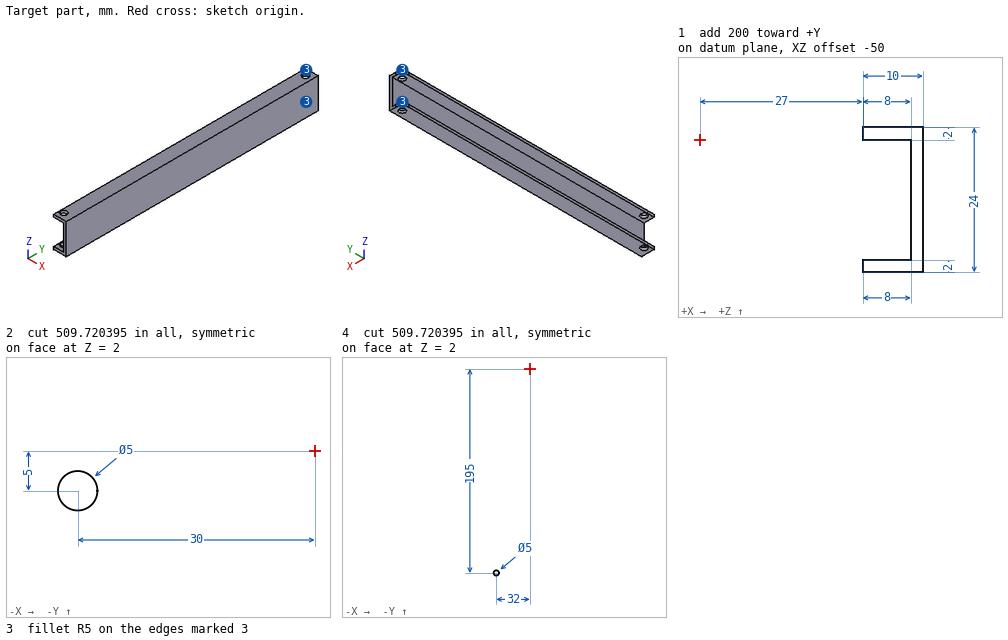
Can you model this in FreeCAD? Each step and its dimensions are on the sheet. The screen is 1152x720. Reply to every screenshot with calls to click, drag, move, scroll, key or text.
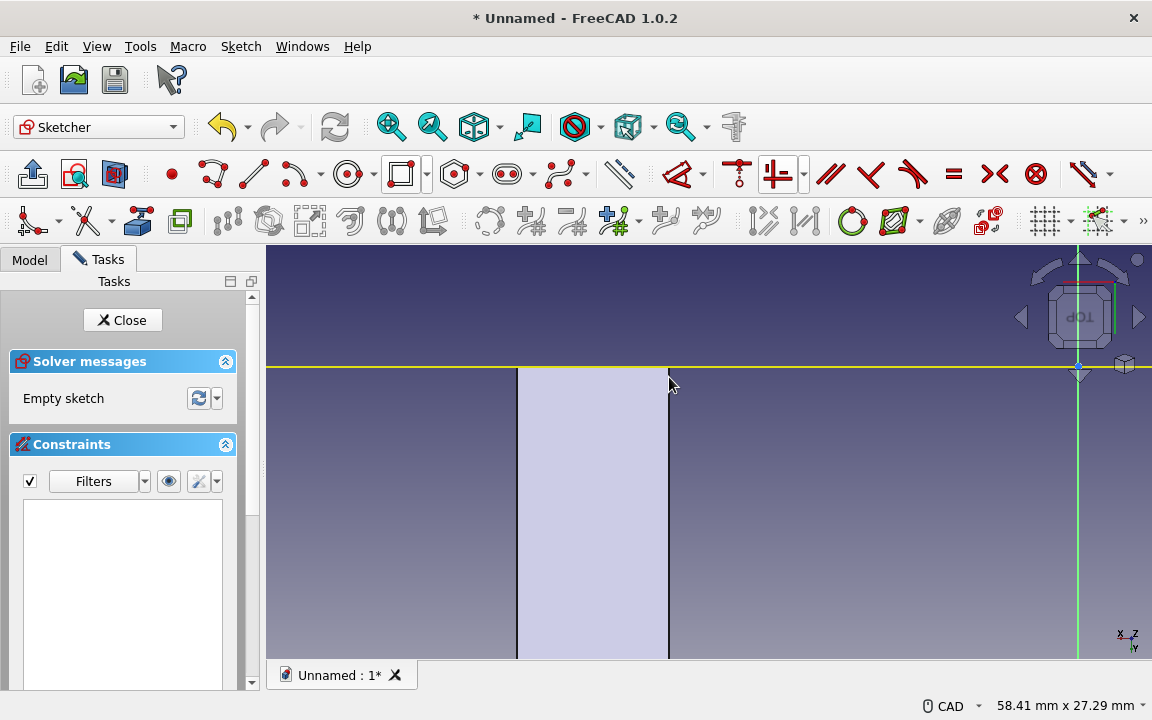
scroll(616, 439, up, 6)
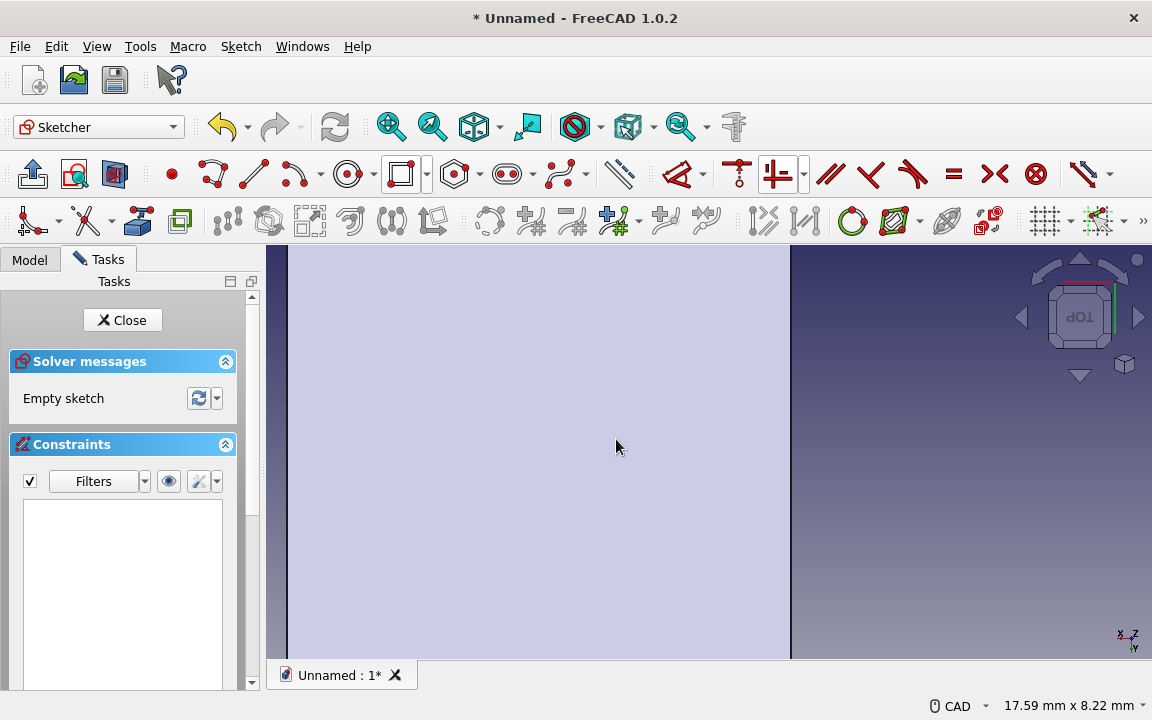
click(348, 174)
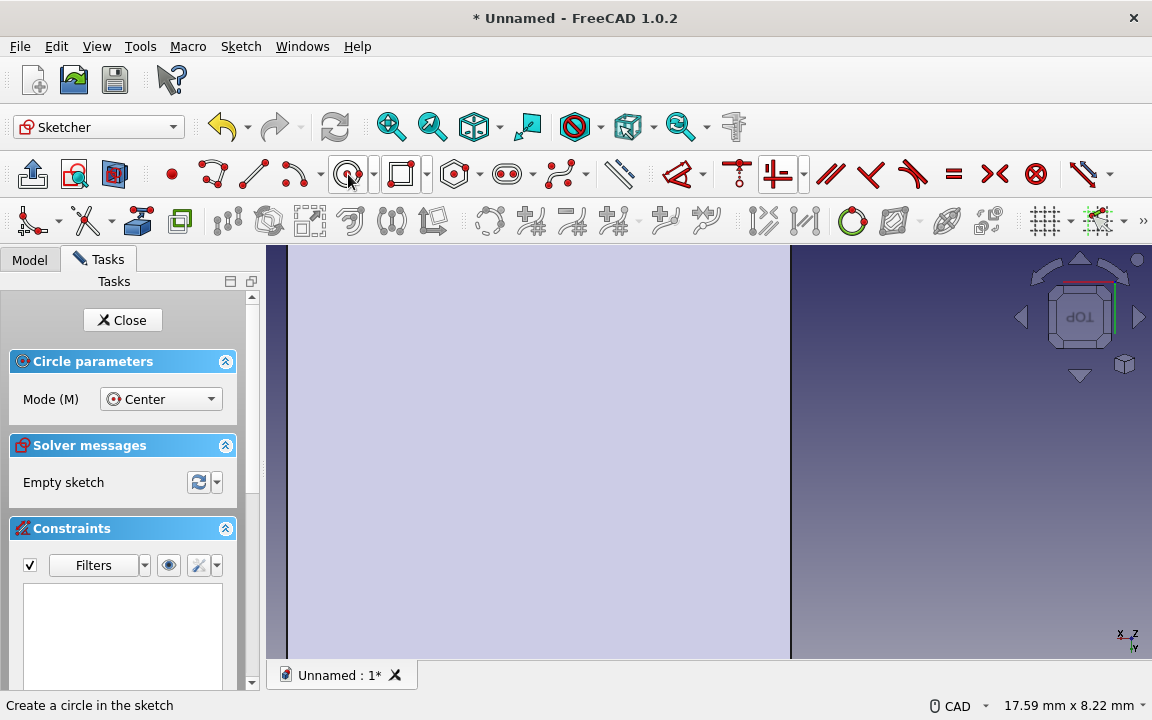
click(640, 450)
move(729, 361)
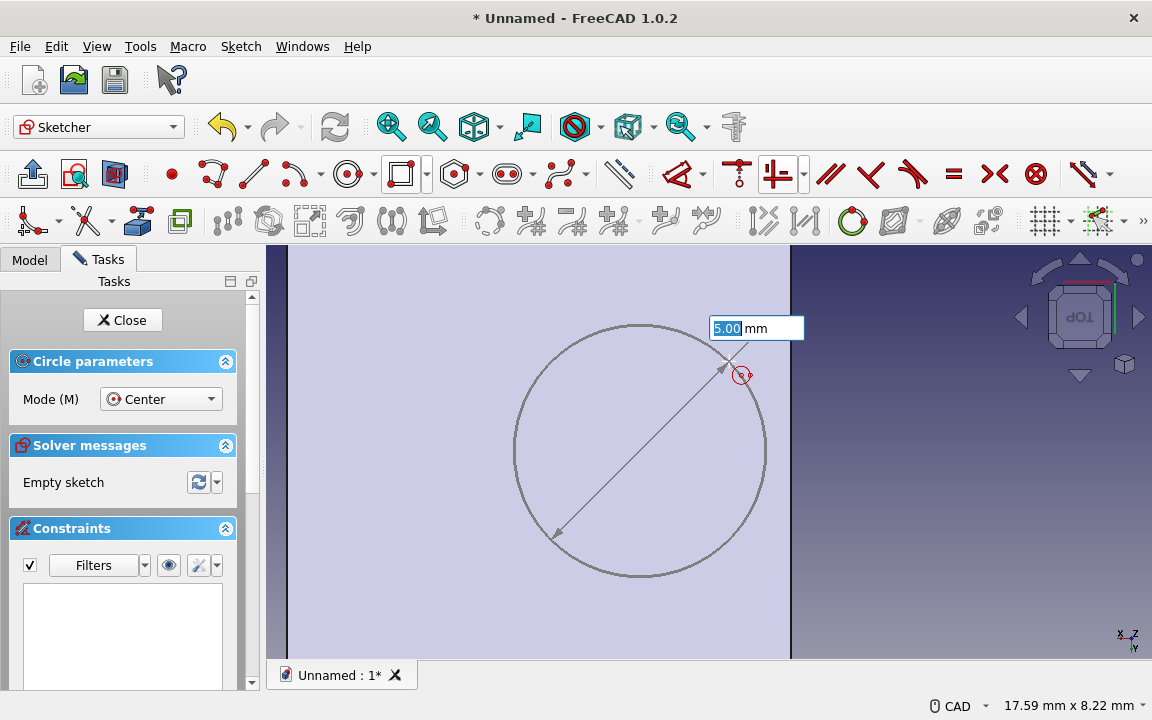
text(5)
key(Return)
key(Escape)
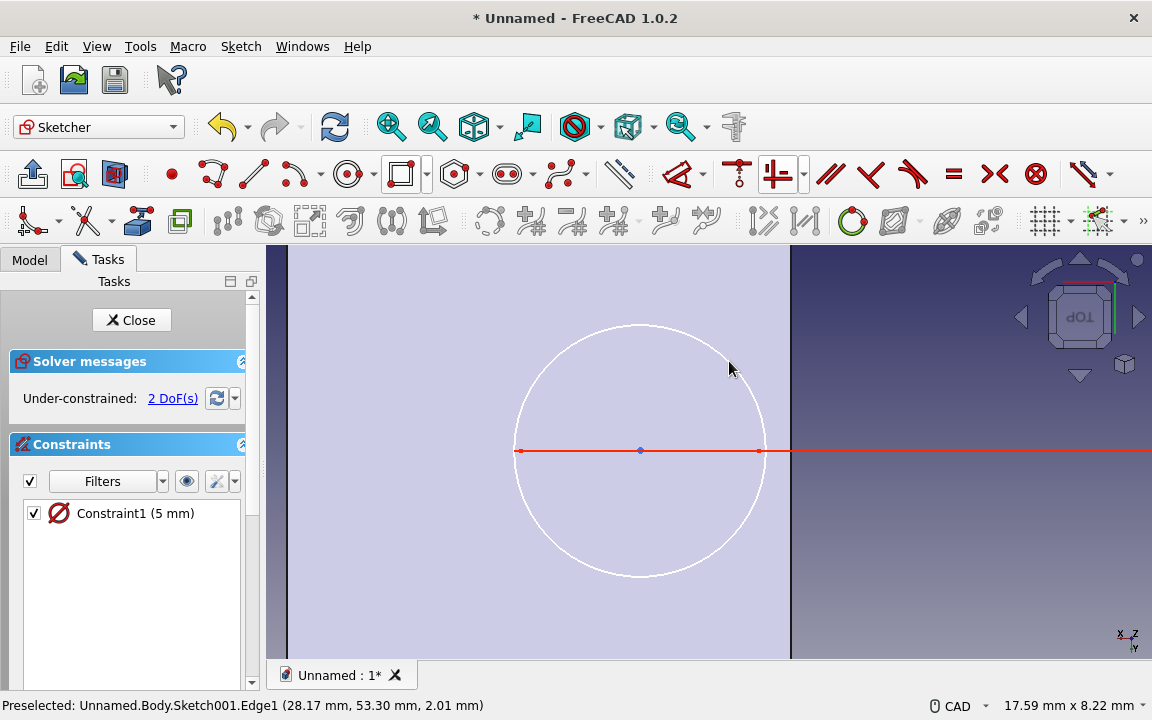
click(676, 174)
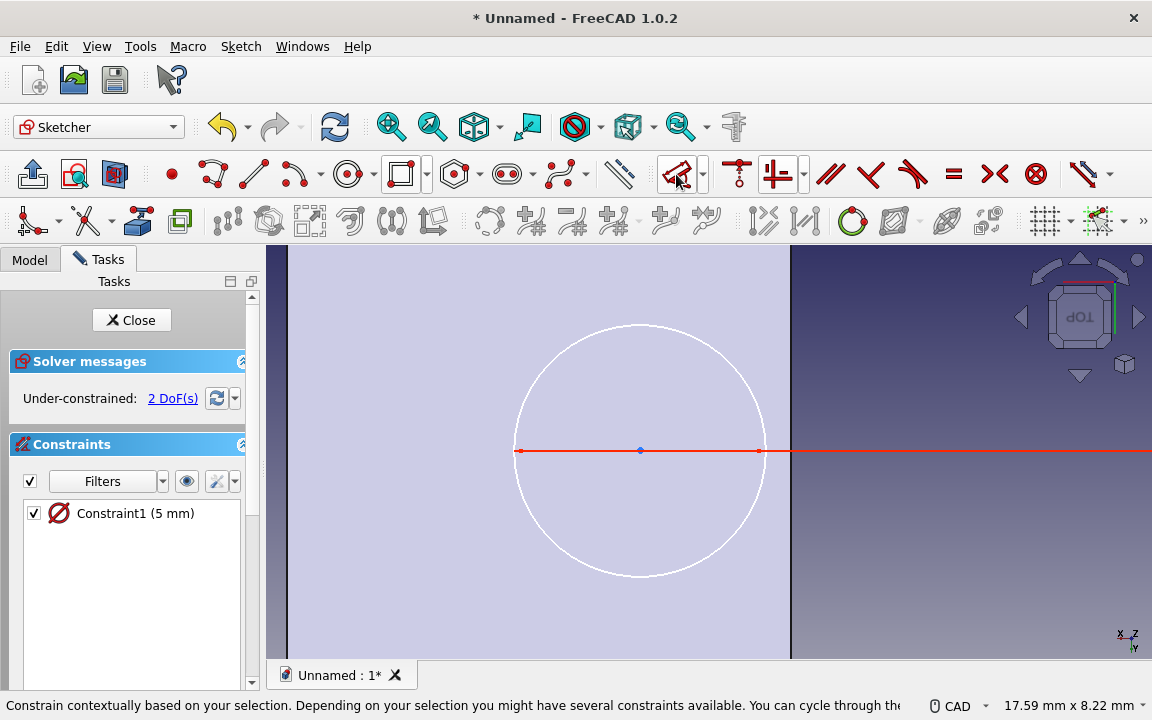
click(640, 451)
click(606, 362)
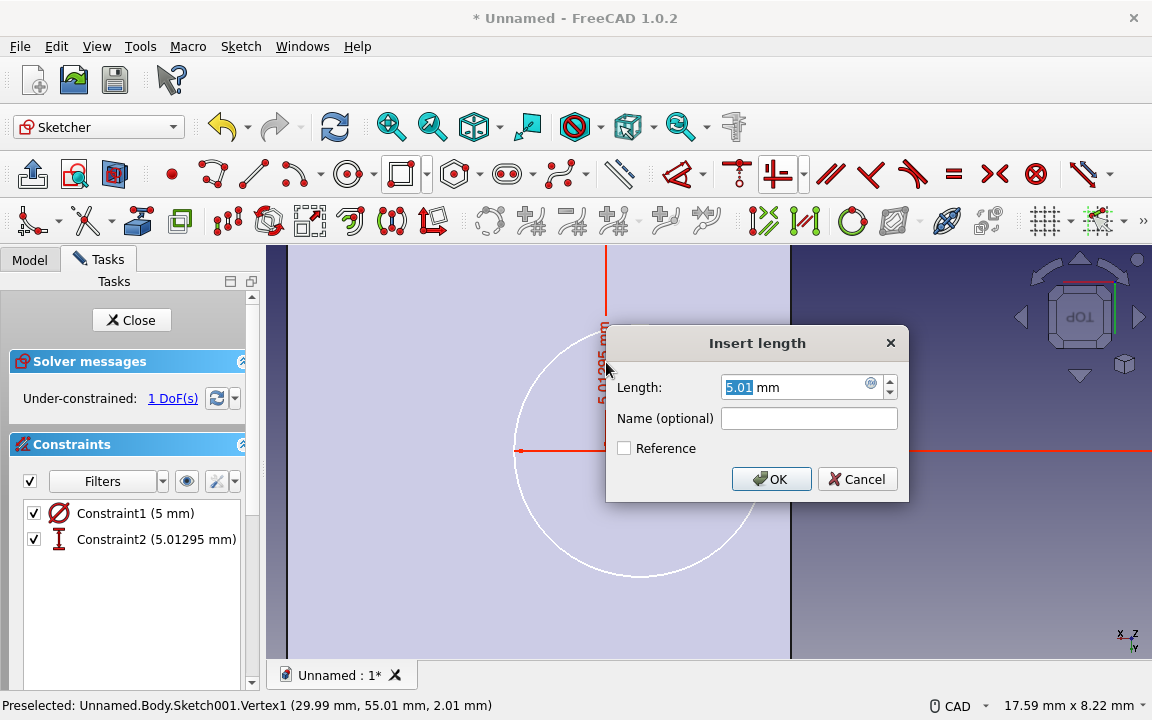
text(5)
key(Return)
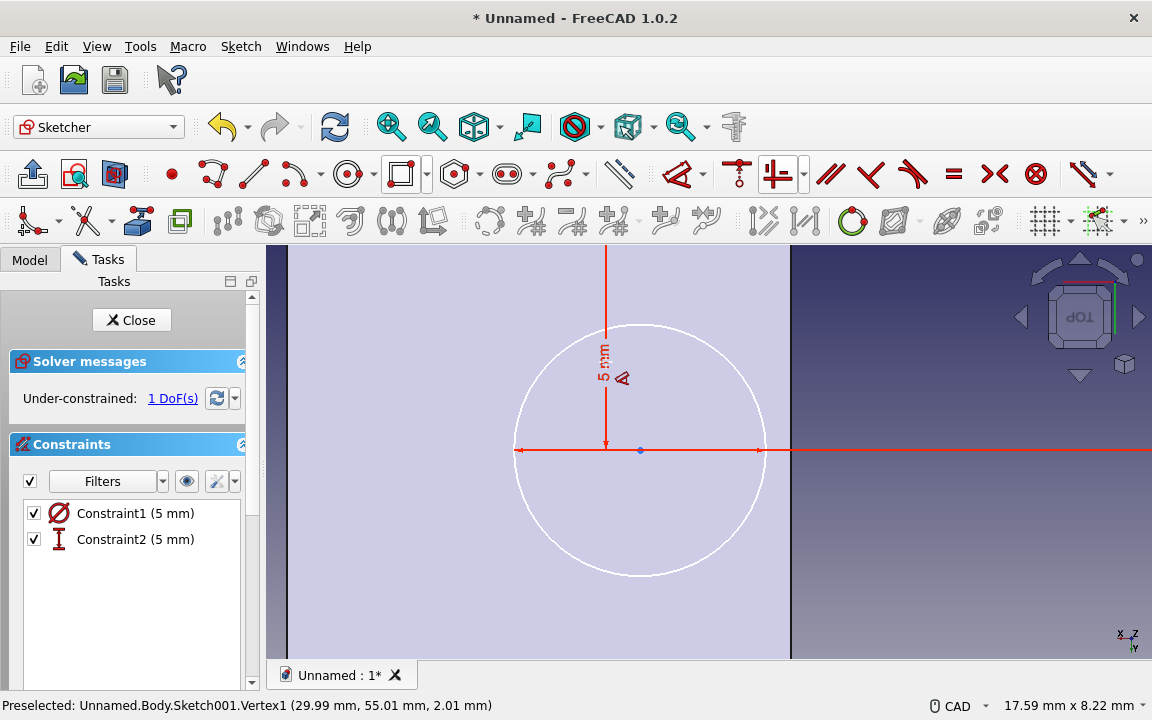
click(640, 450)
click(813, 484)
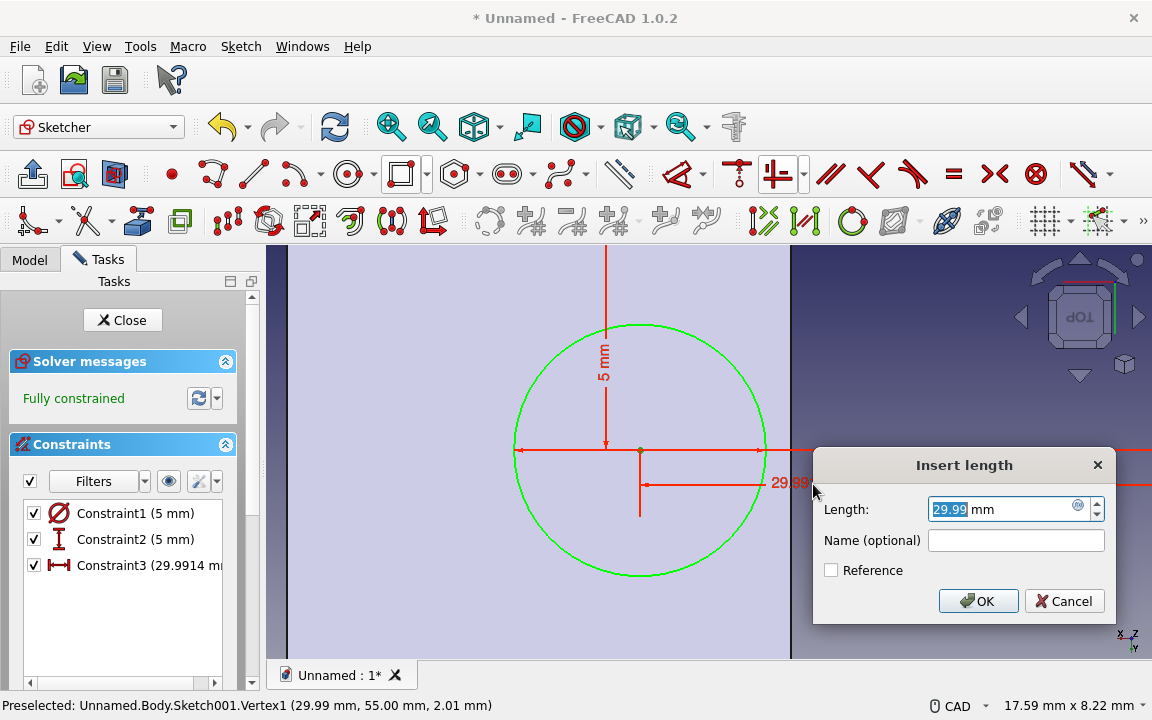
text(30)
key(Return)
key(Escape)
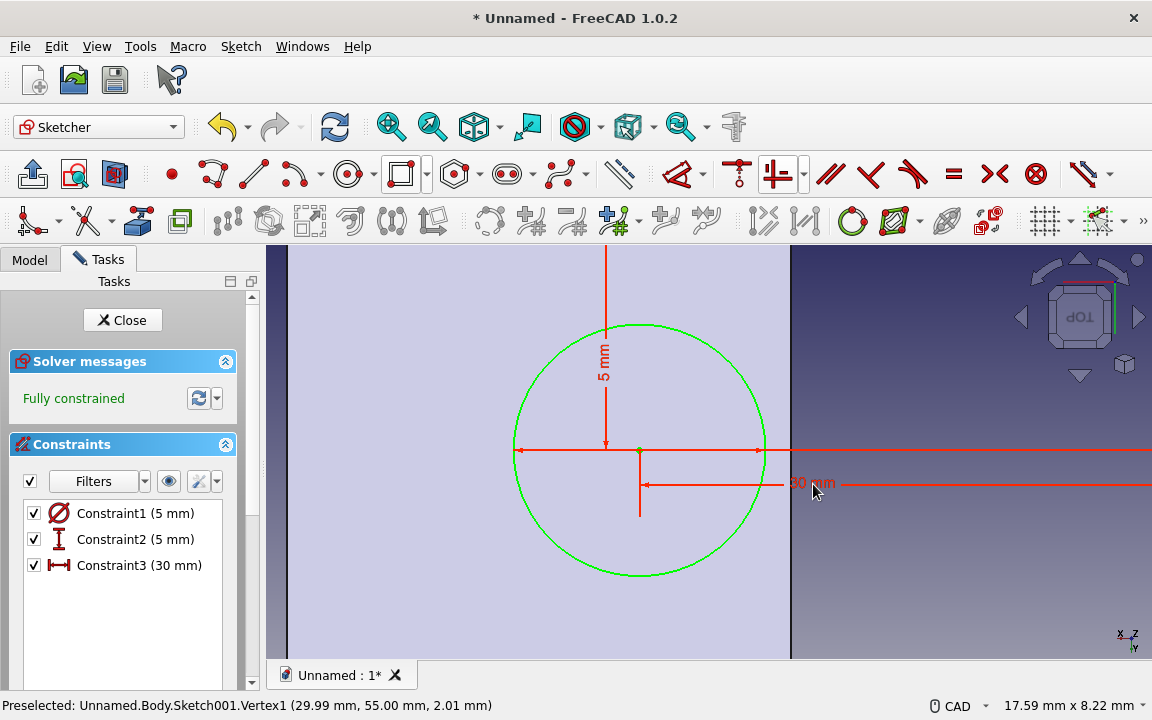
click(123, 320)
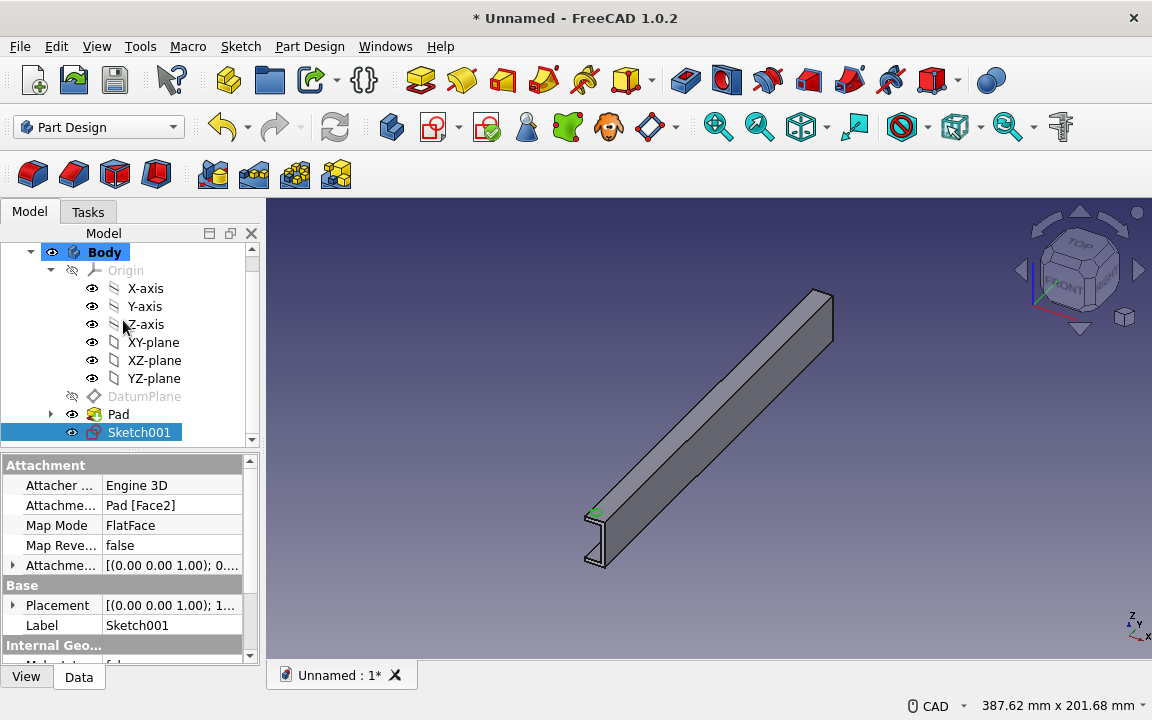
click(686, 80)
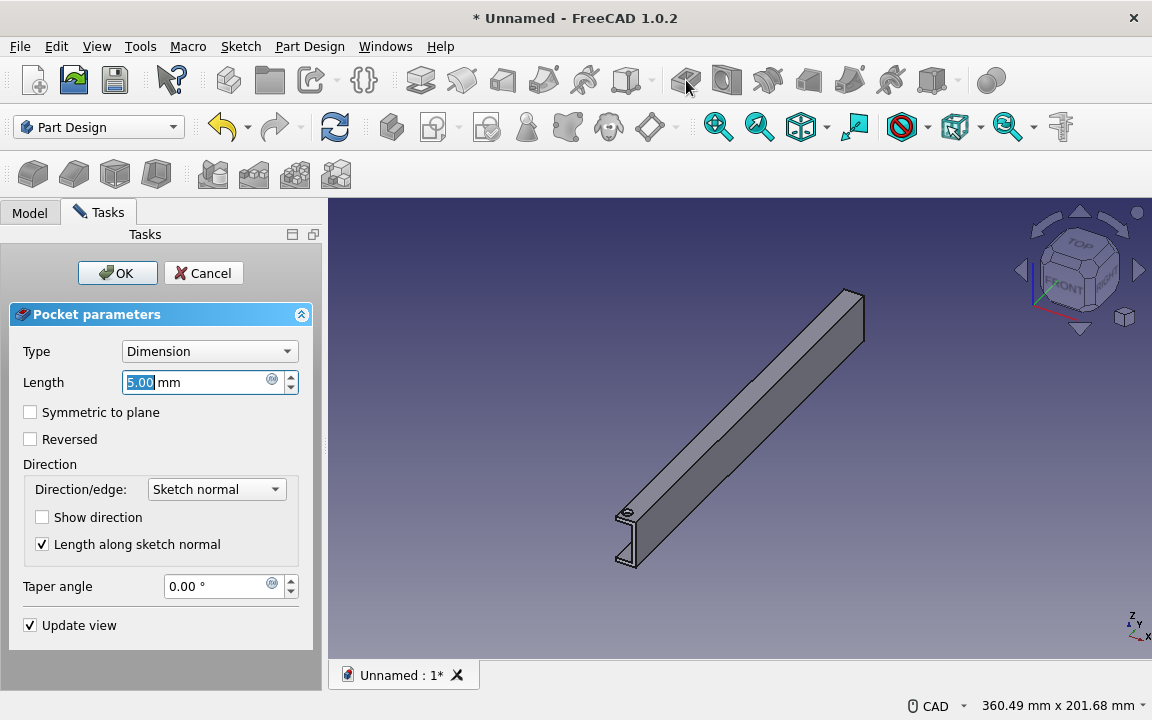
text(509.720395)
key(Tab)